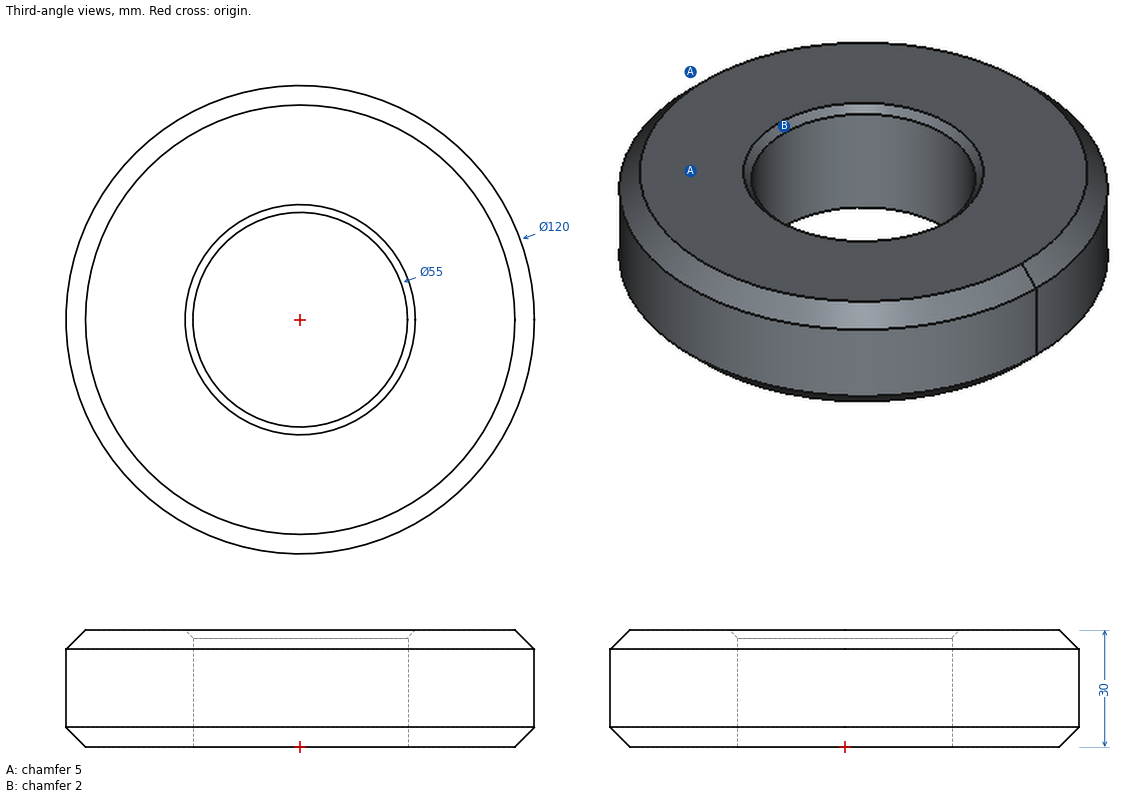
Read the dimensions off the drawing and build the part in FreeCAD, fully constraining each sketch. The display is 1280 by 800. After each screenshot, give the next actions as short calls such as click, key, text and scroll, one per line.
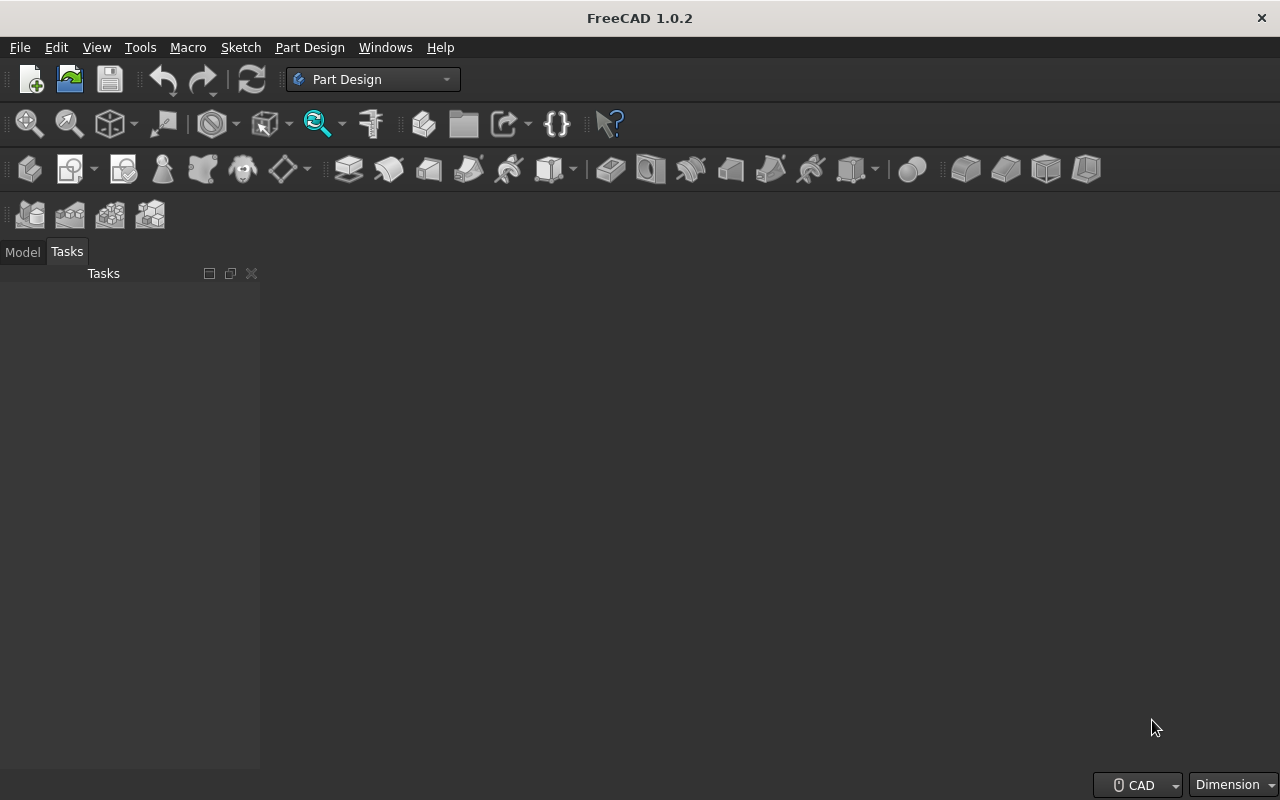
click(30, 80)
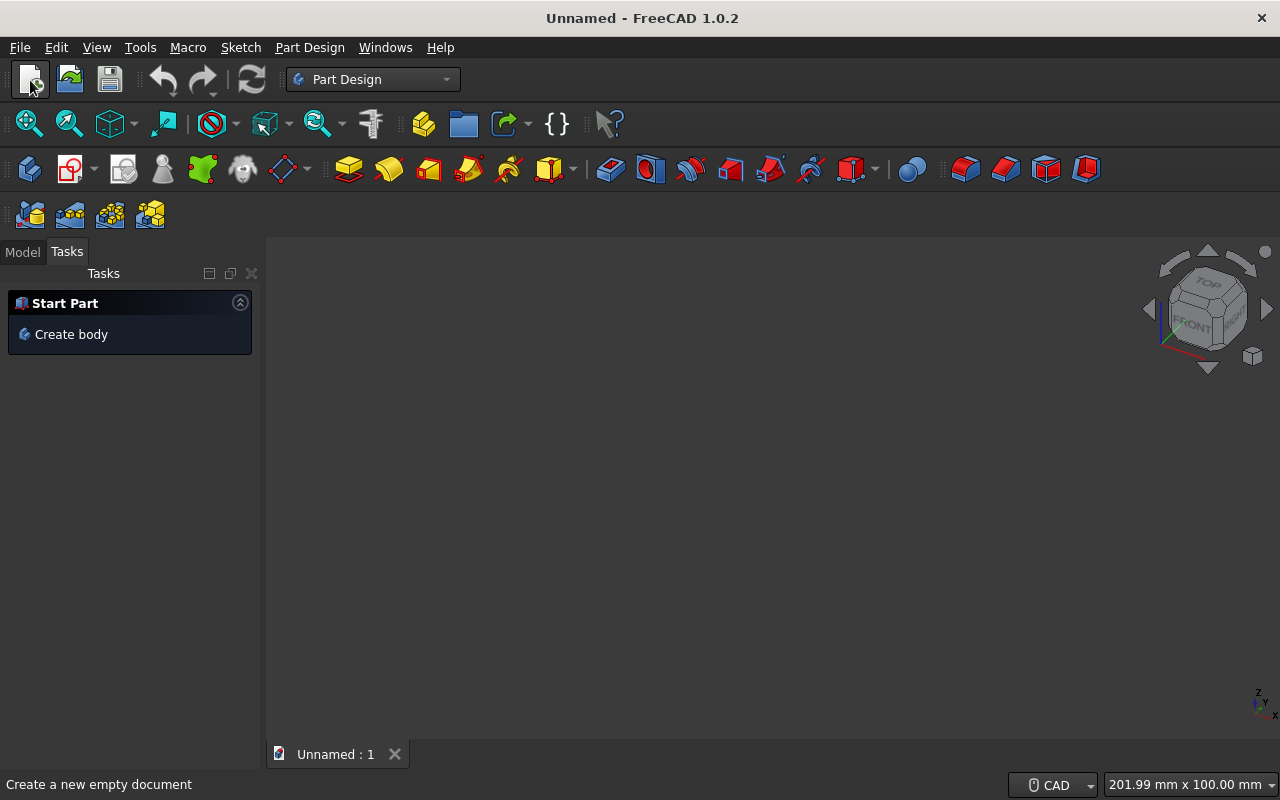
click(70, 170)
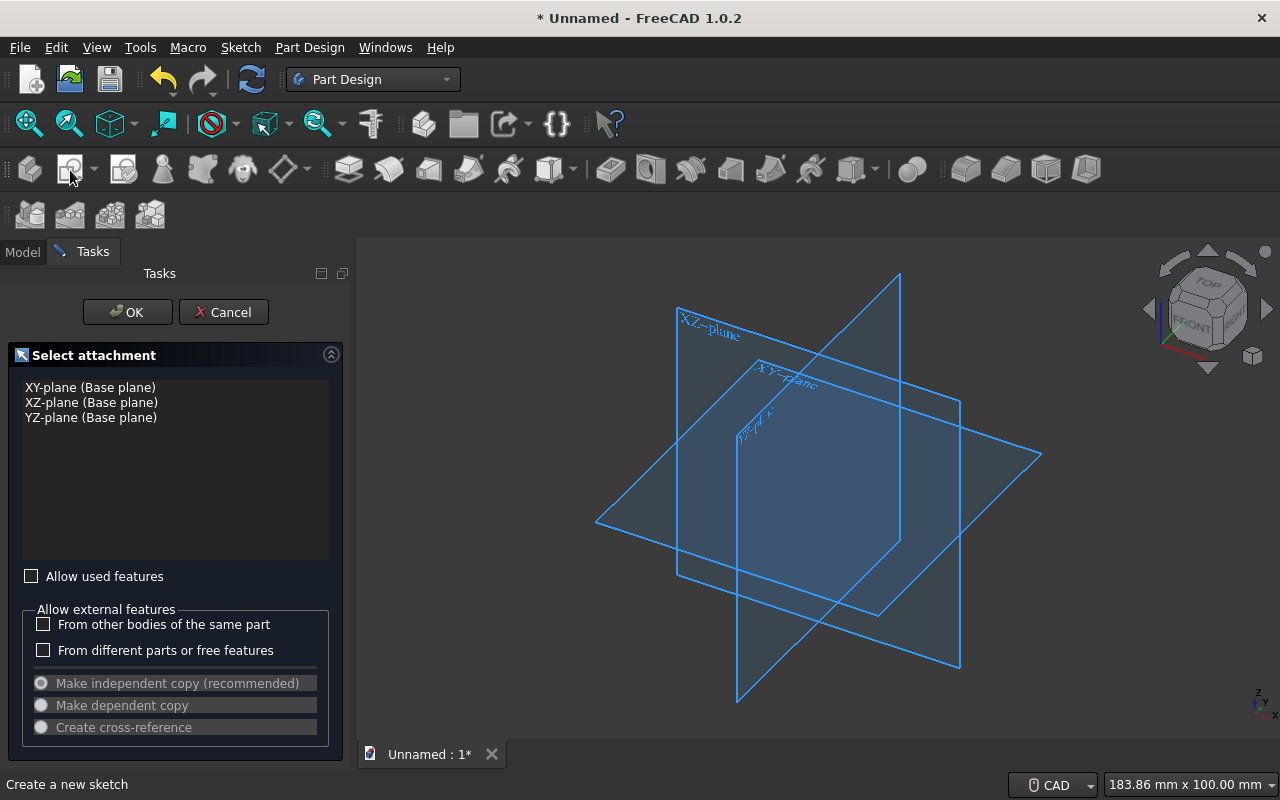
click(82, 388)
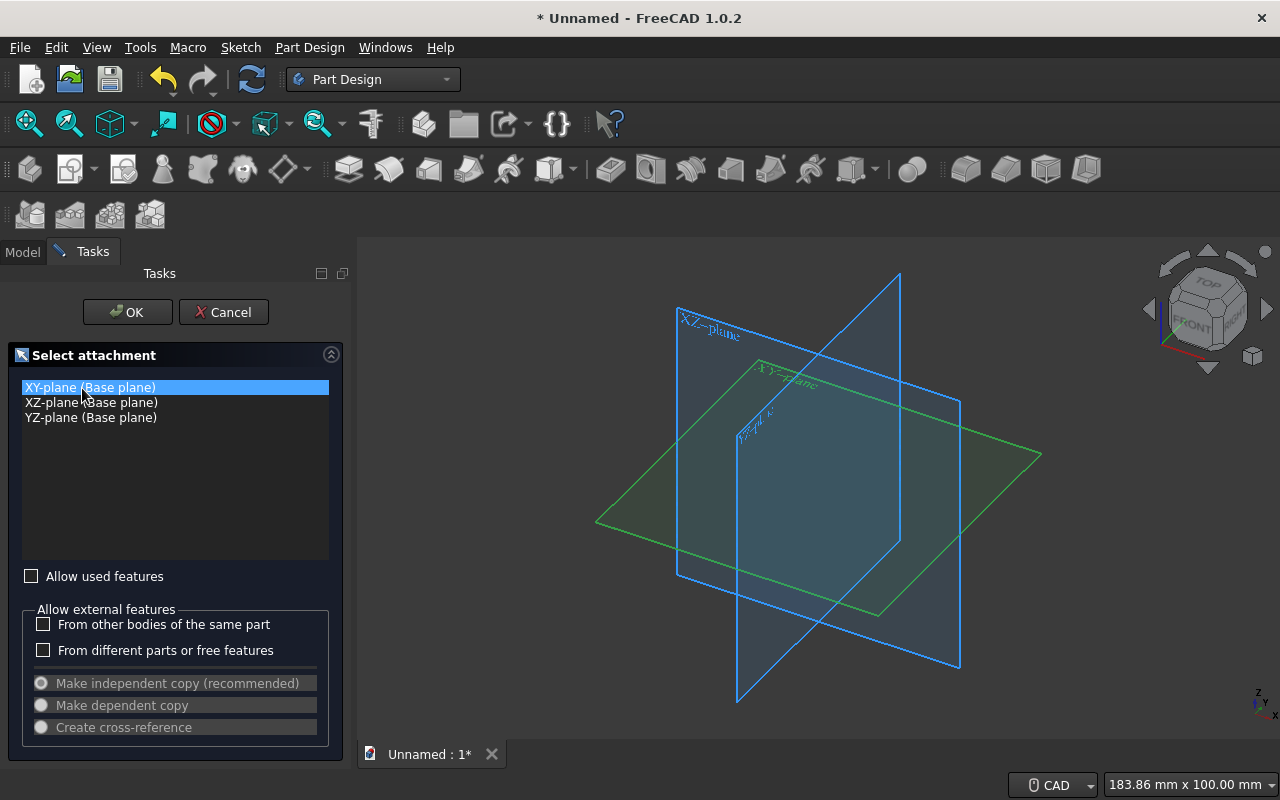
click(128, 312)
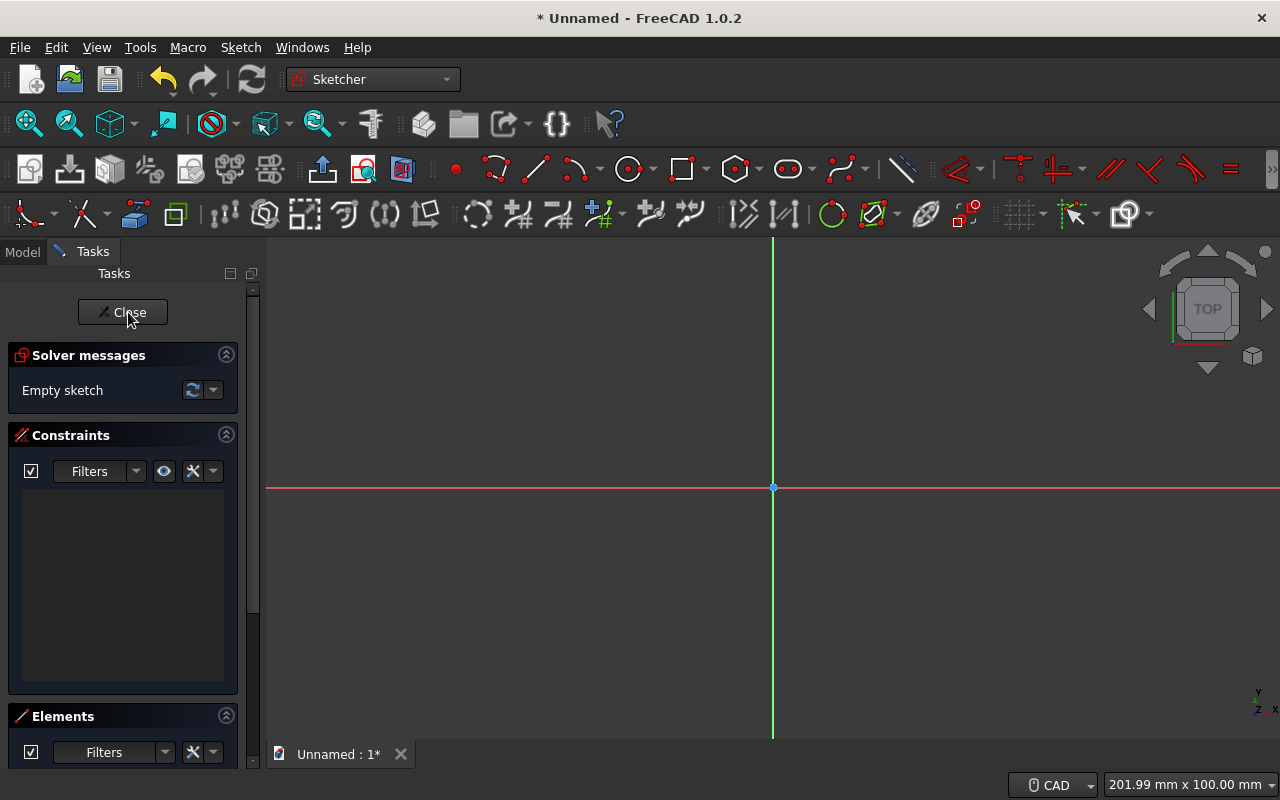
scroll(621, 488, down, 3)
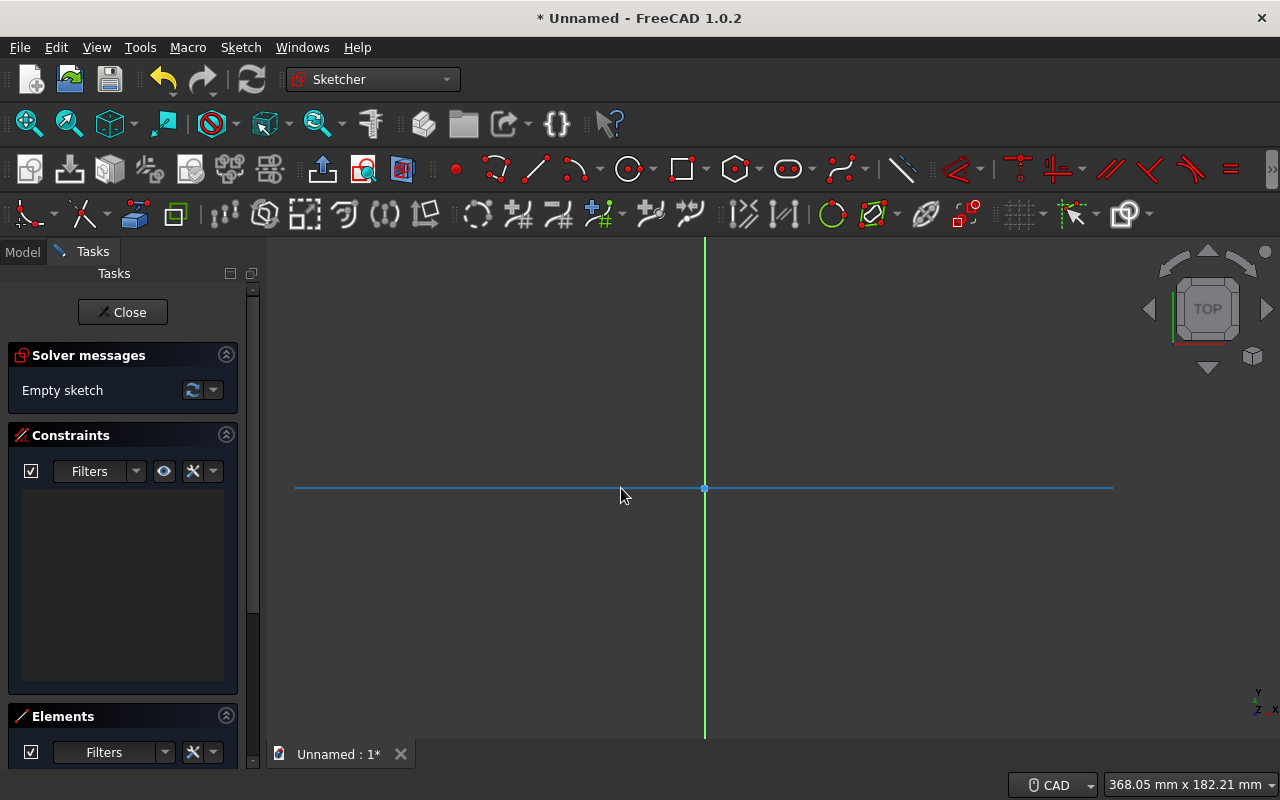
click(630, 170)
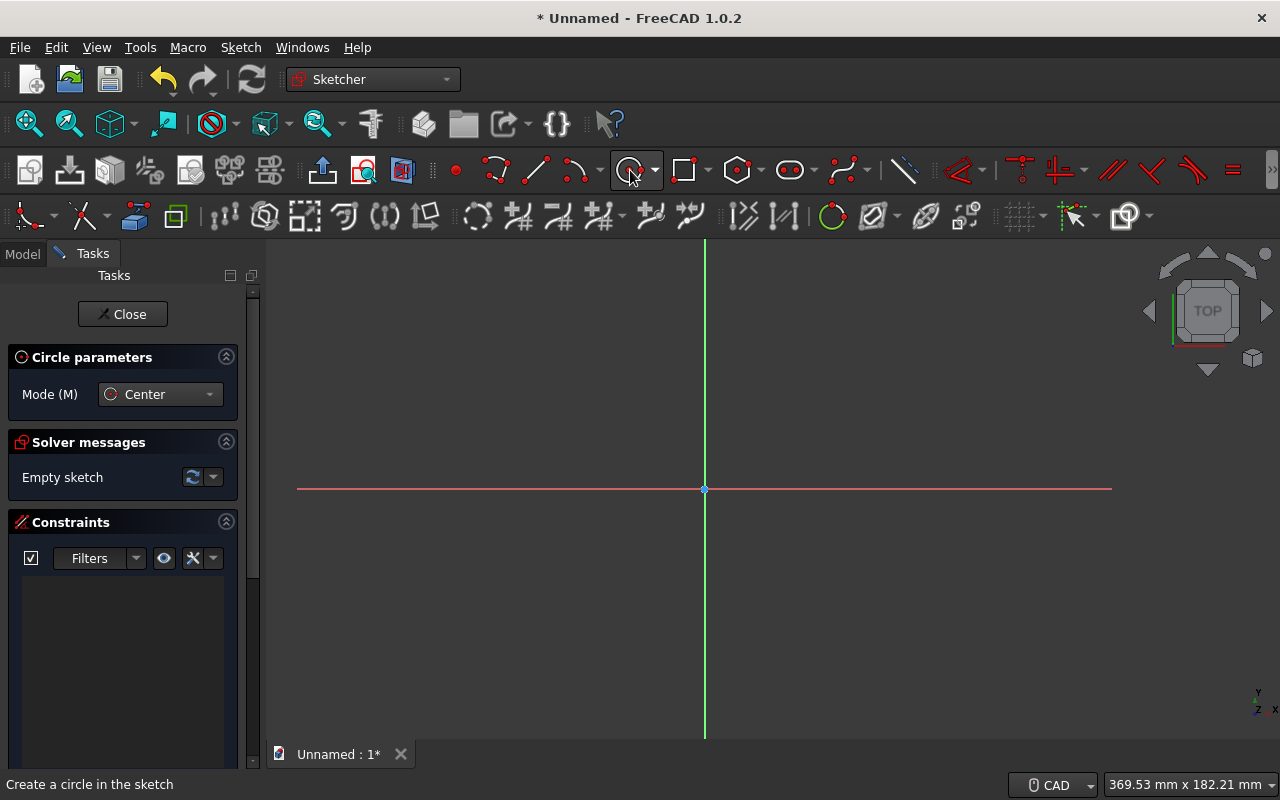
click(705, 489)
move(821, 373)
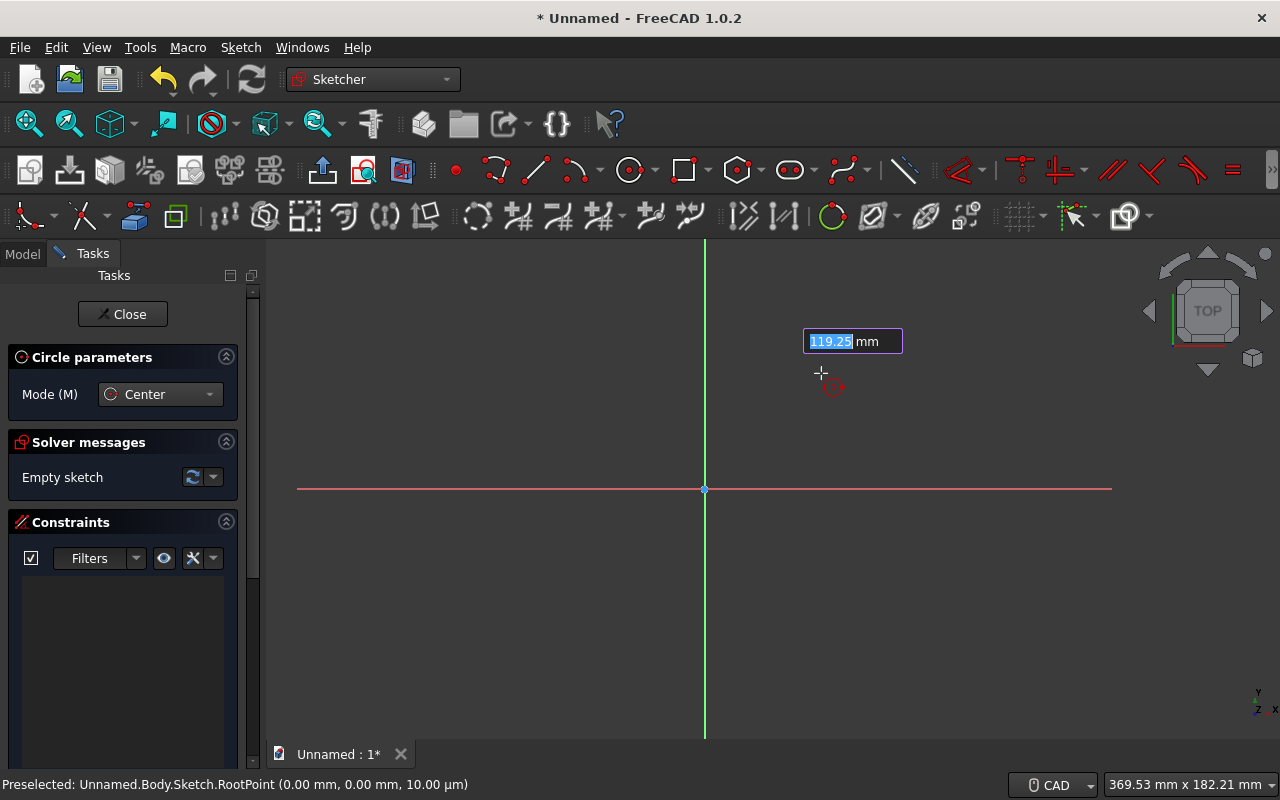
text(120)
key(Return)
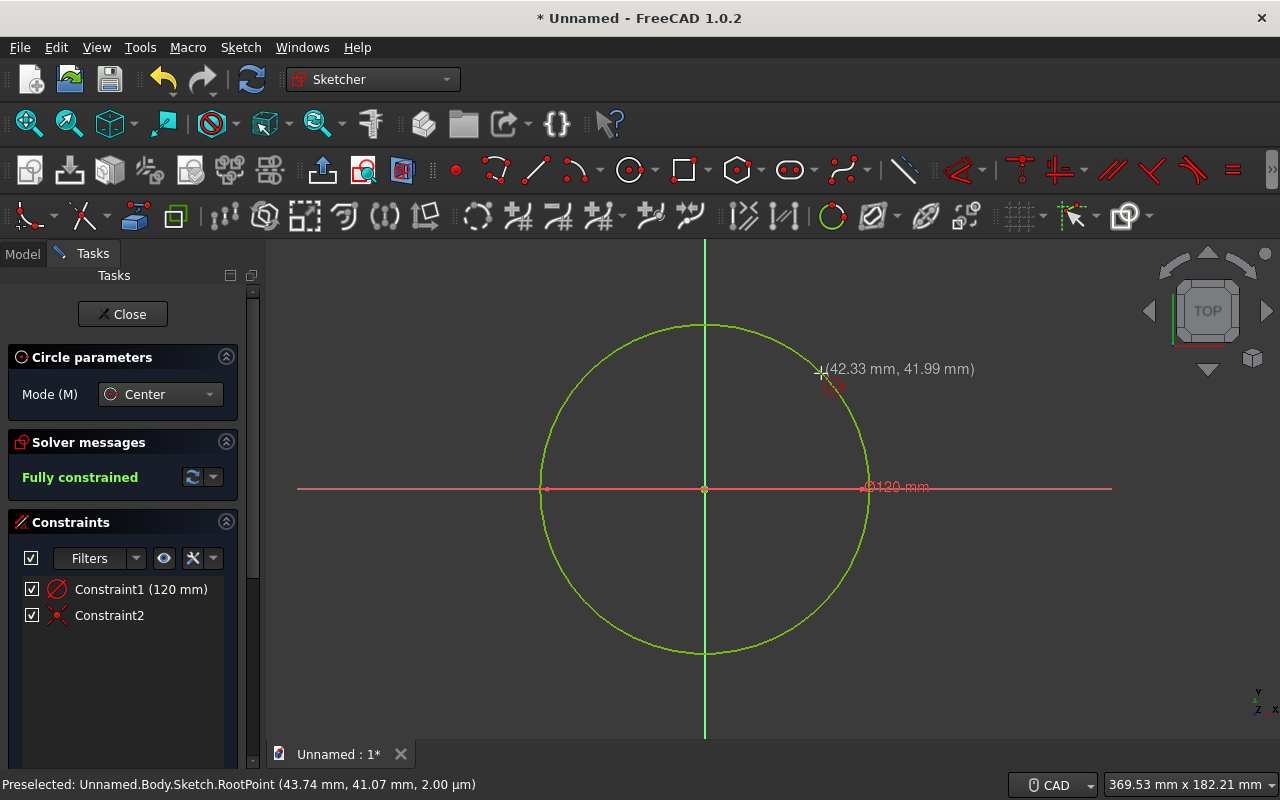
click(705, 489)
move(758, 436)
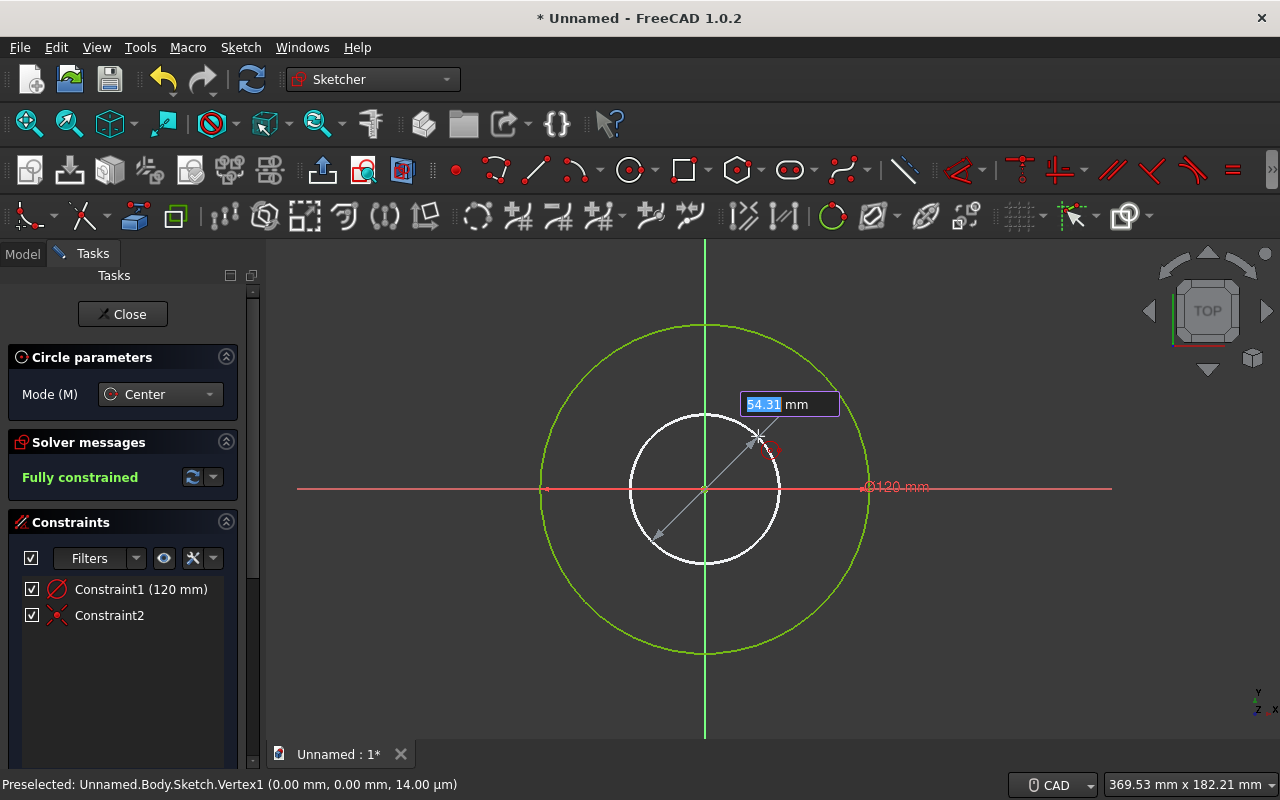
text(55)
key(Return)
key(Escape)